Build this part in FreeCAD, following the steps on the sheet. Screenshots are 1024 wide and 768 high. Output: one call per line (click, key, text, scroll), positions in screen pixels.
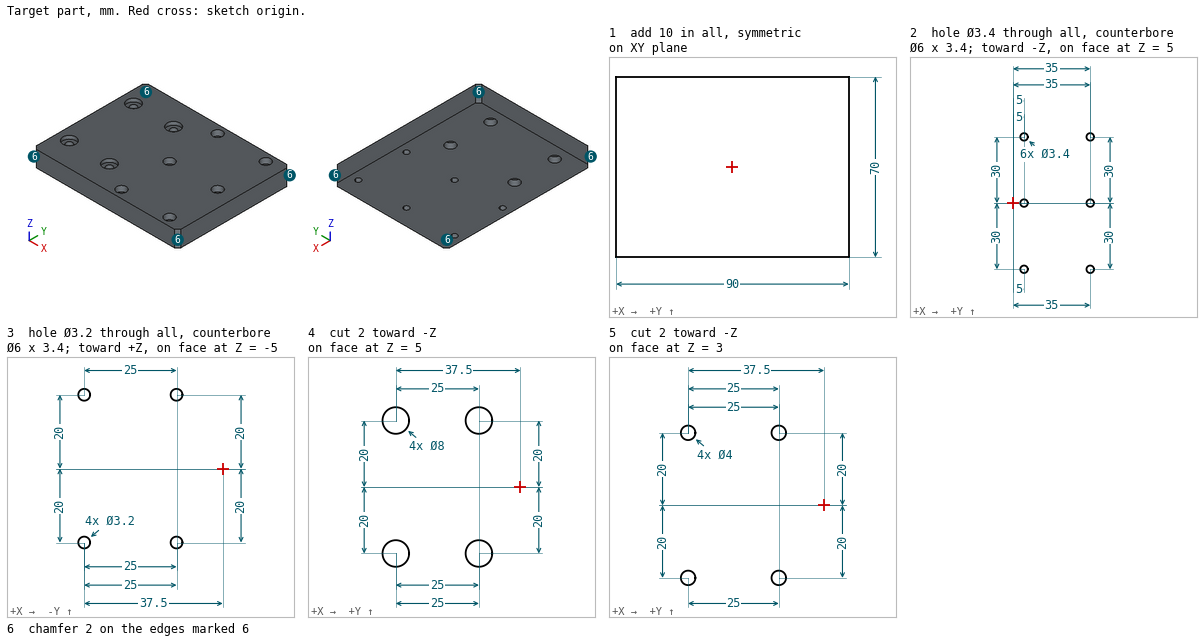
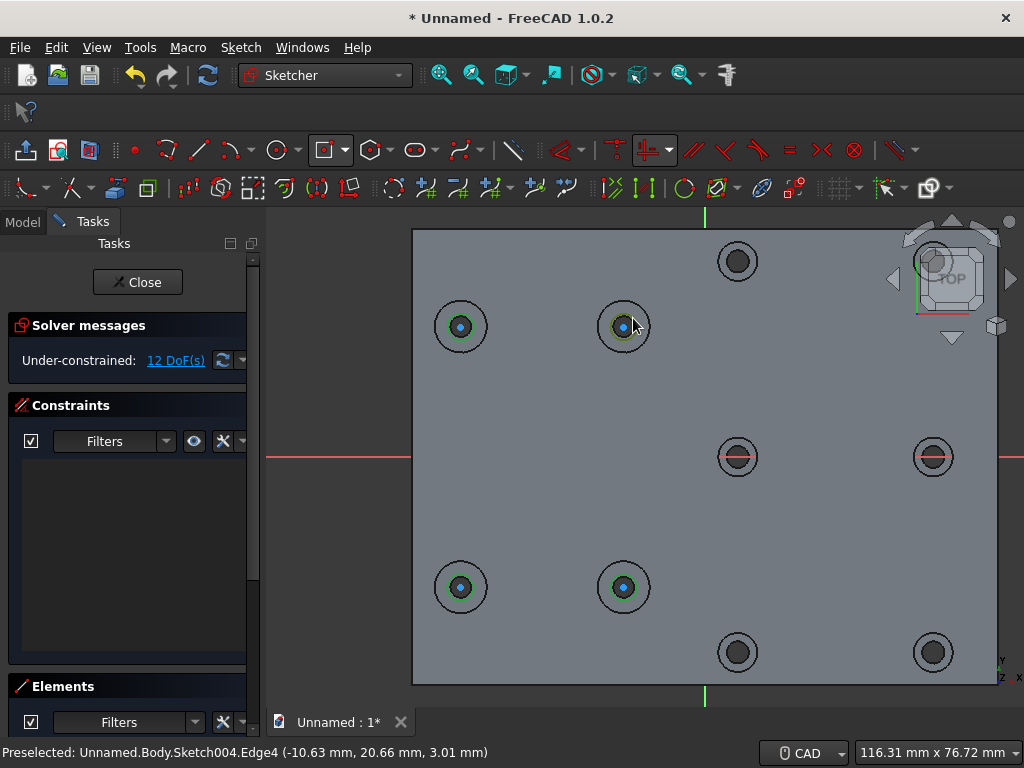
click(790, 150)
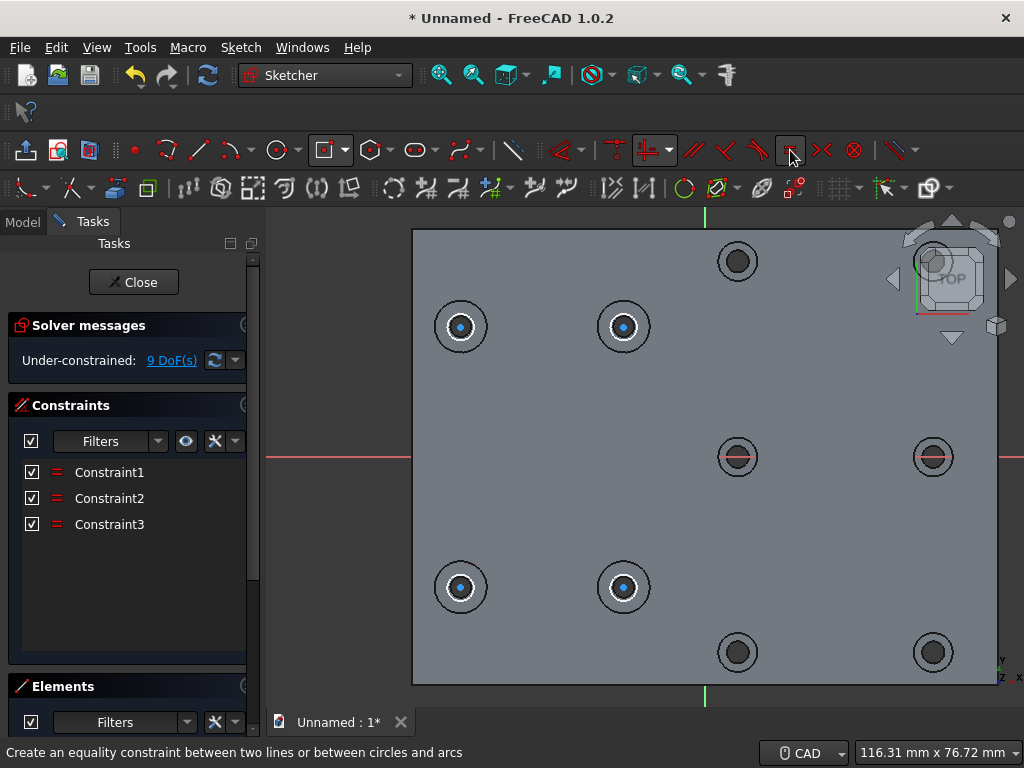
click(560, 150)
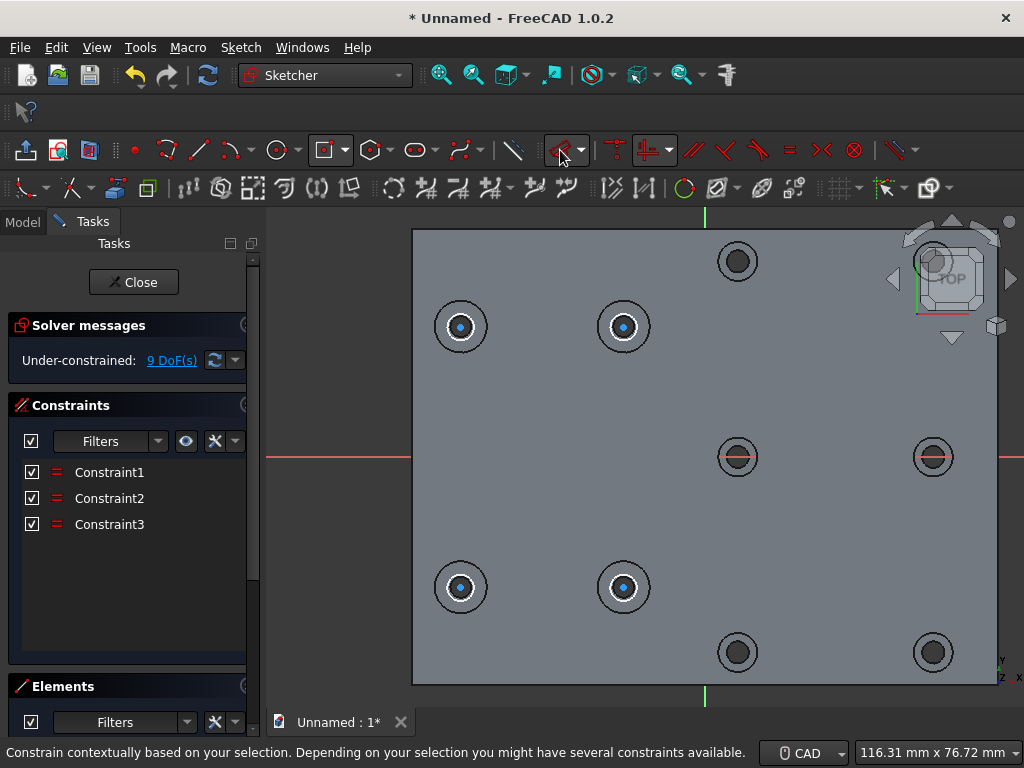
scroll(470, 318, up, 3)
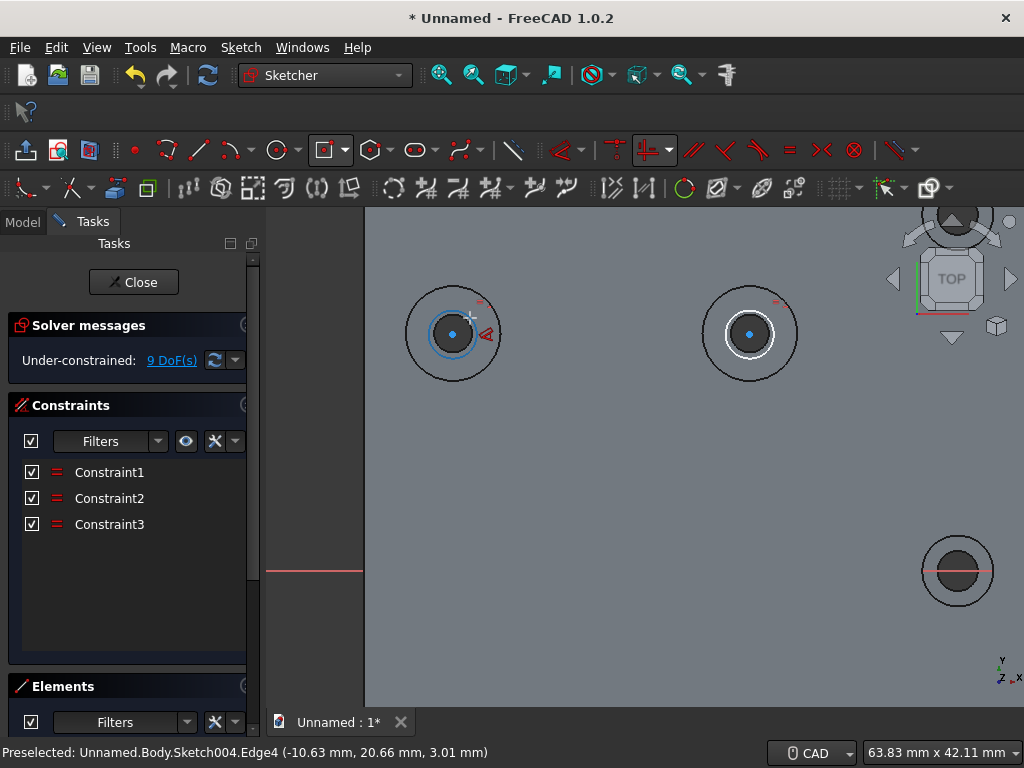
click(470, 318)
click(493, 296)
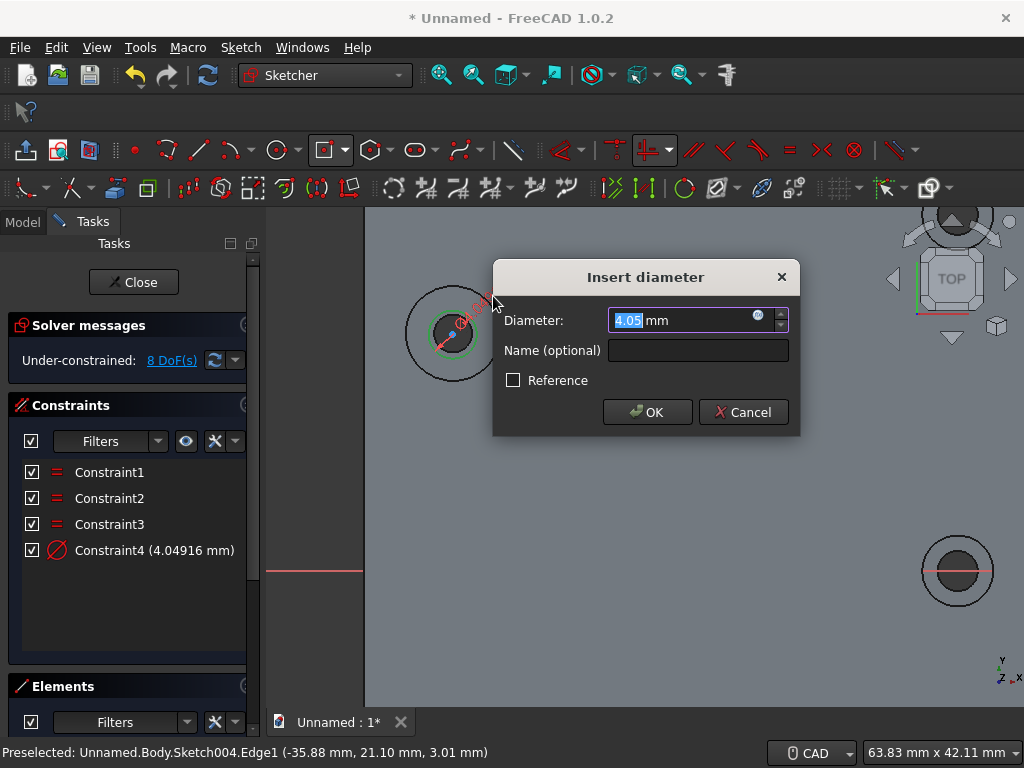
text(4)
key(Return)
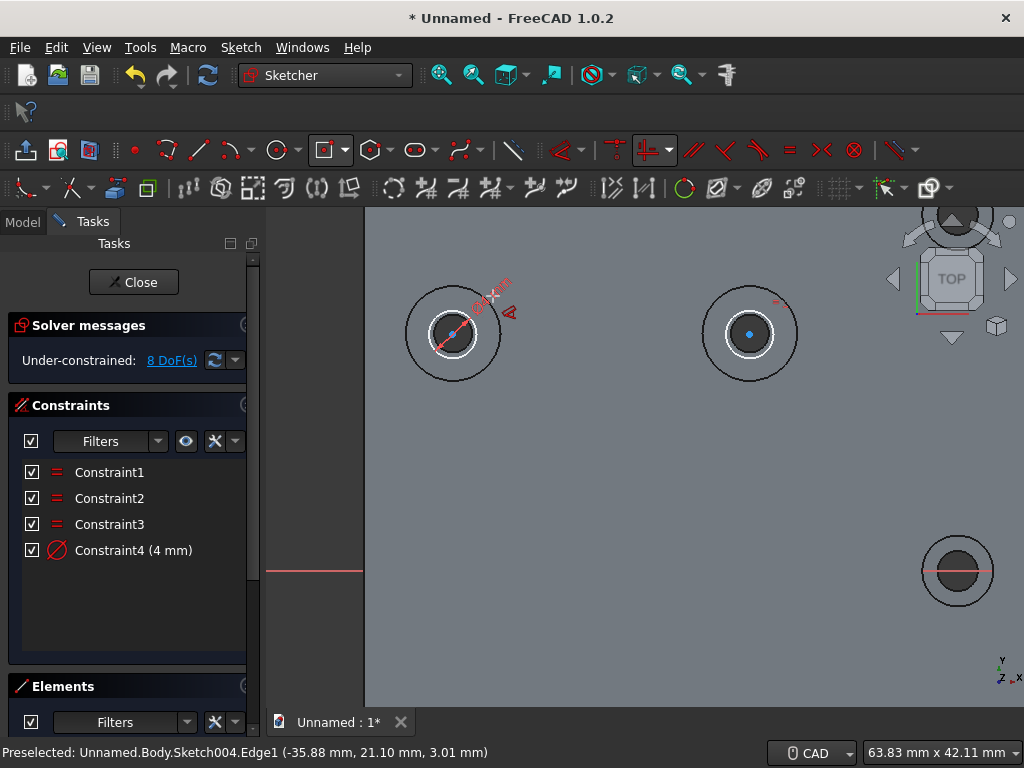
click(453, 335)
click(419, 453)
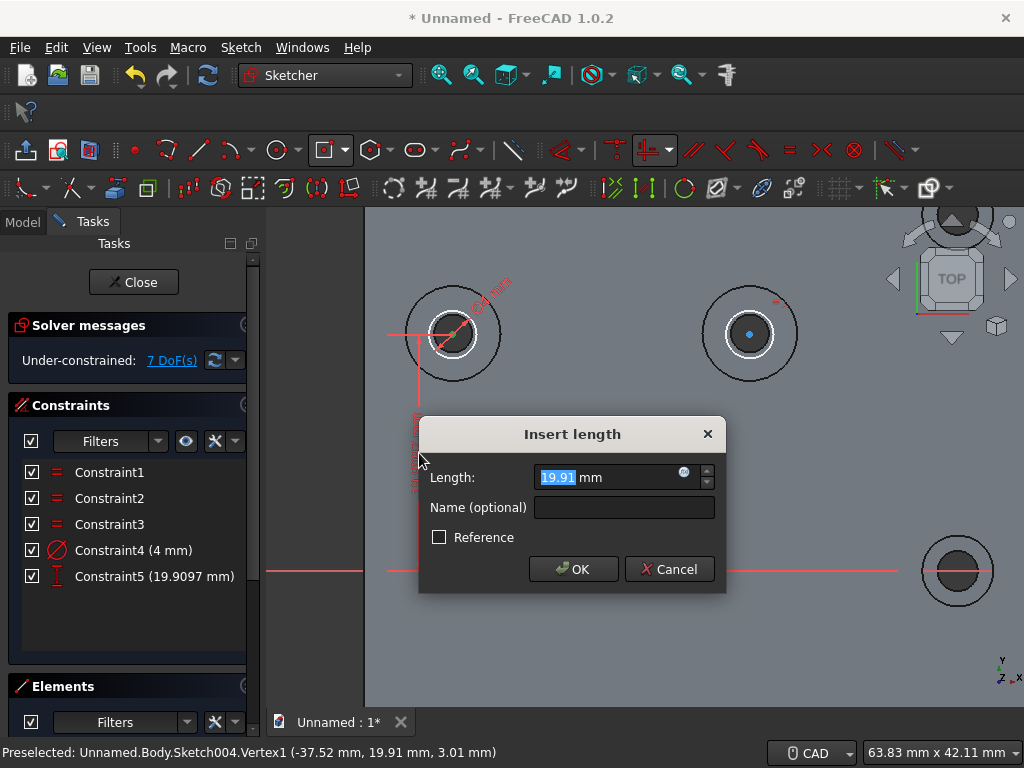
text(20)
key(Return)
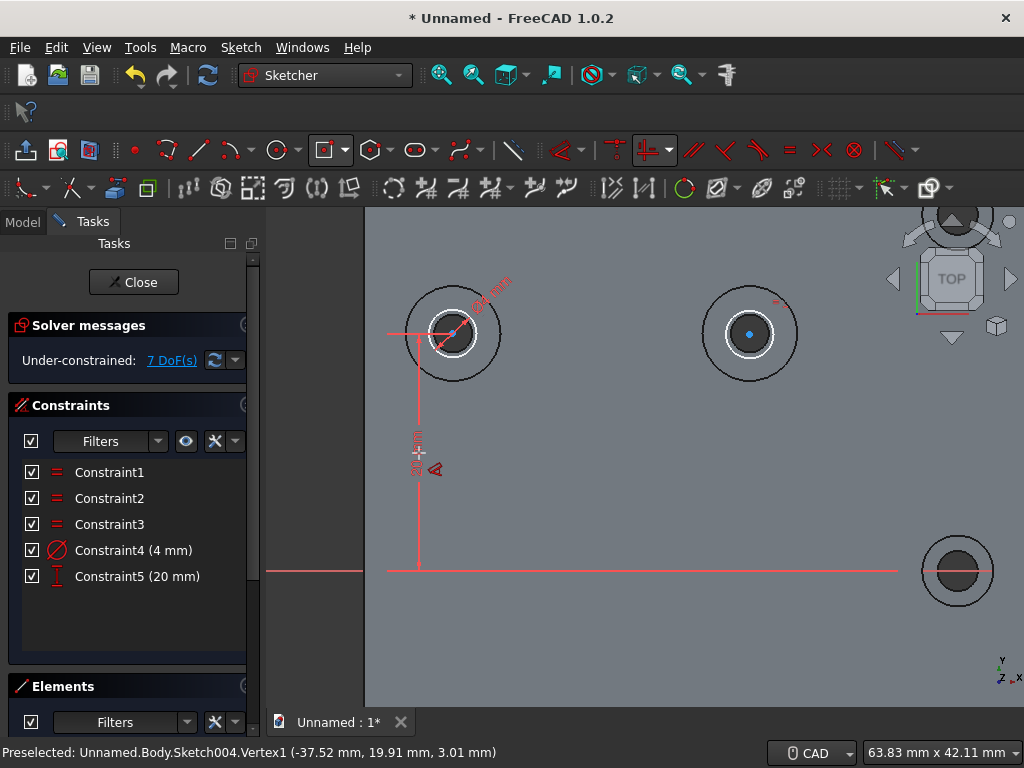
scroll(470, 318, down, 3)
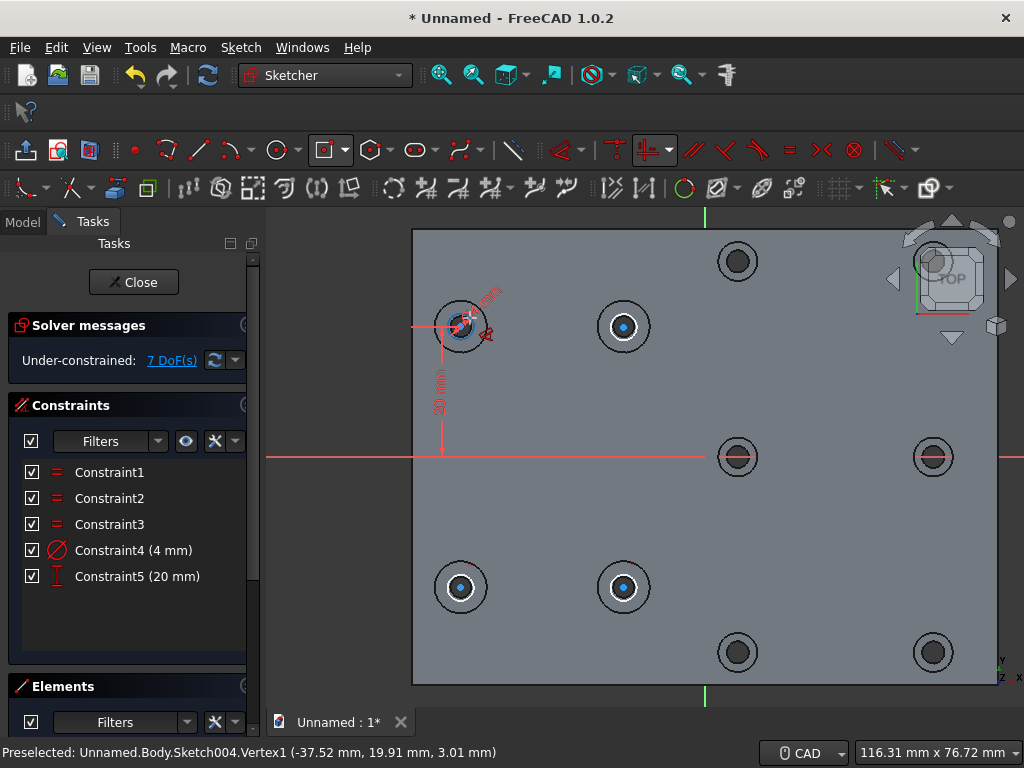
click(461, 588)
click(739, 522)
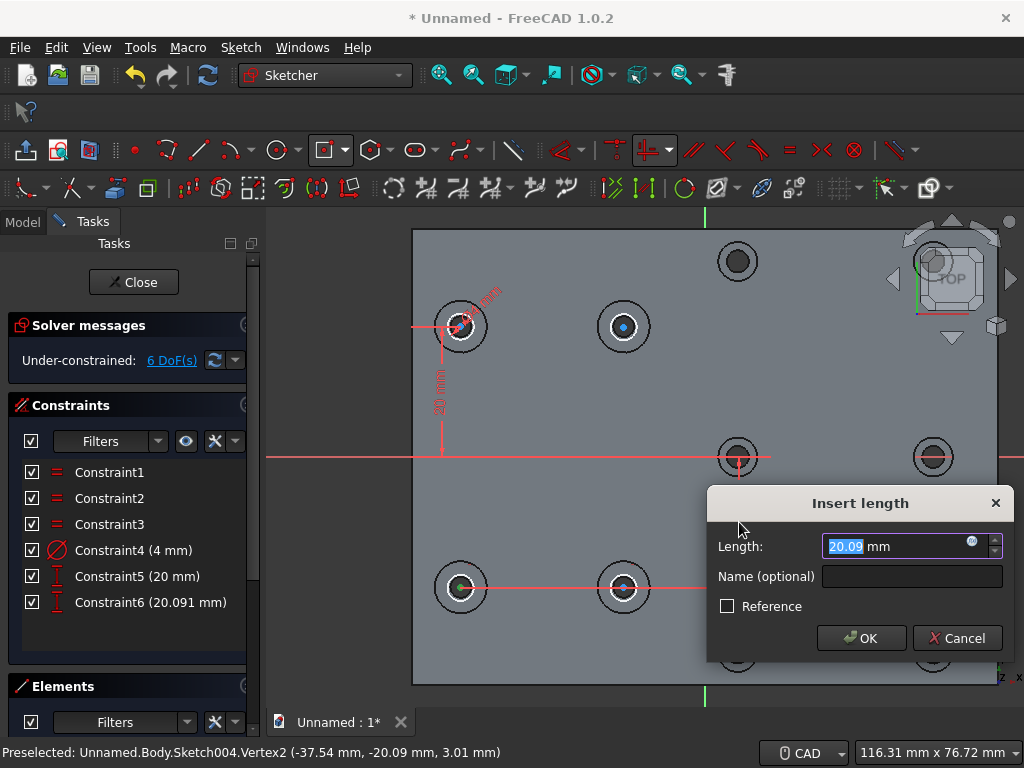
text(20)
key(Return)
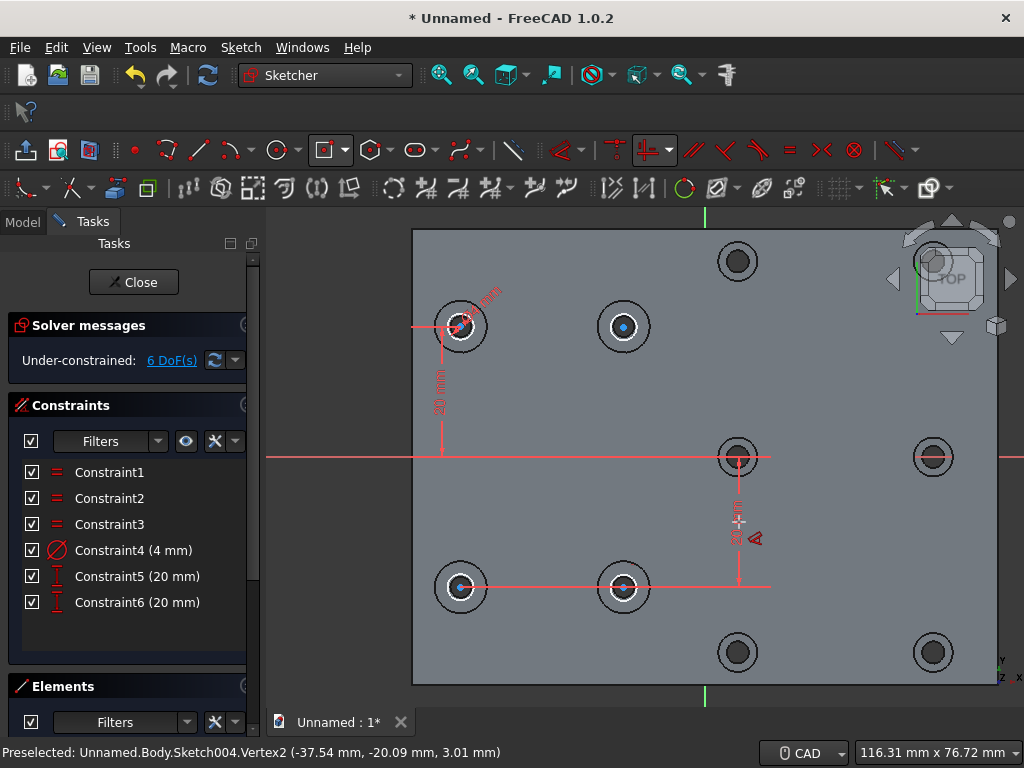
click(624, 588)
click(739, 492)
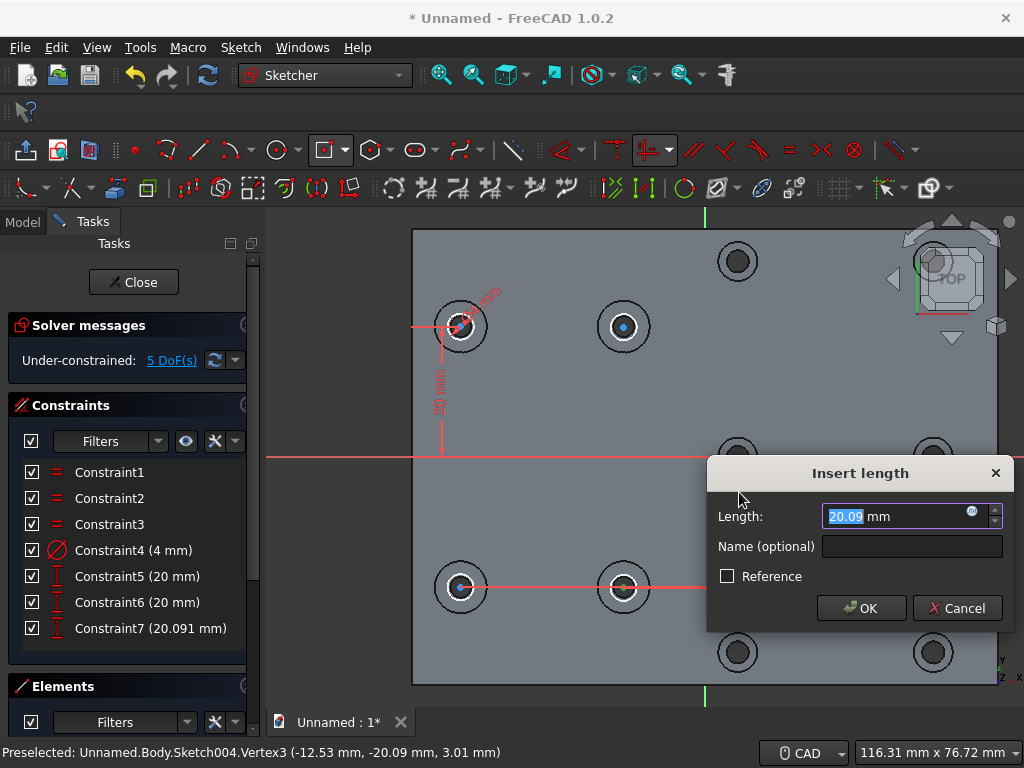
text(20)
key(Return)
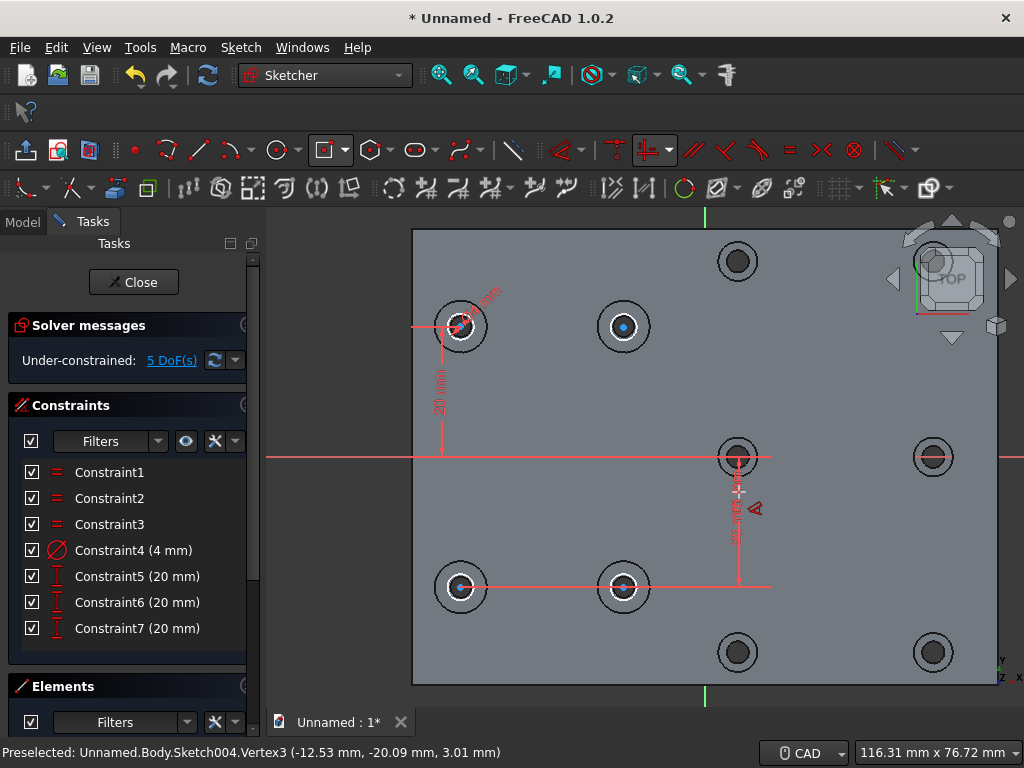
click(624, 327)
click(739, 392)